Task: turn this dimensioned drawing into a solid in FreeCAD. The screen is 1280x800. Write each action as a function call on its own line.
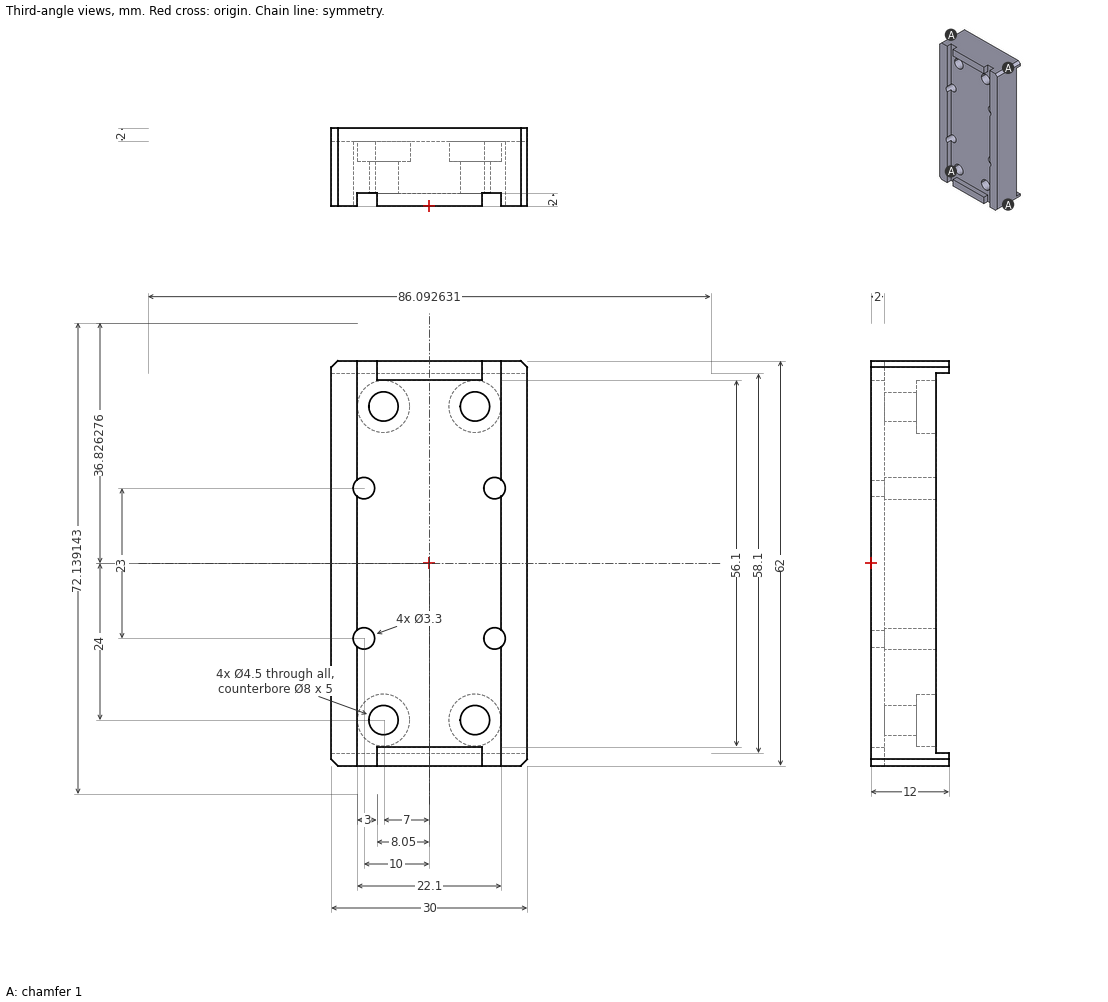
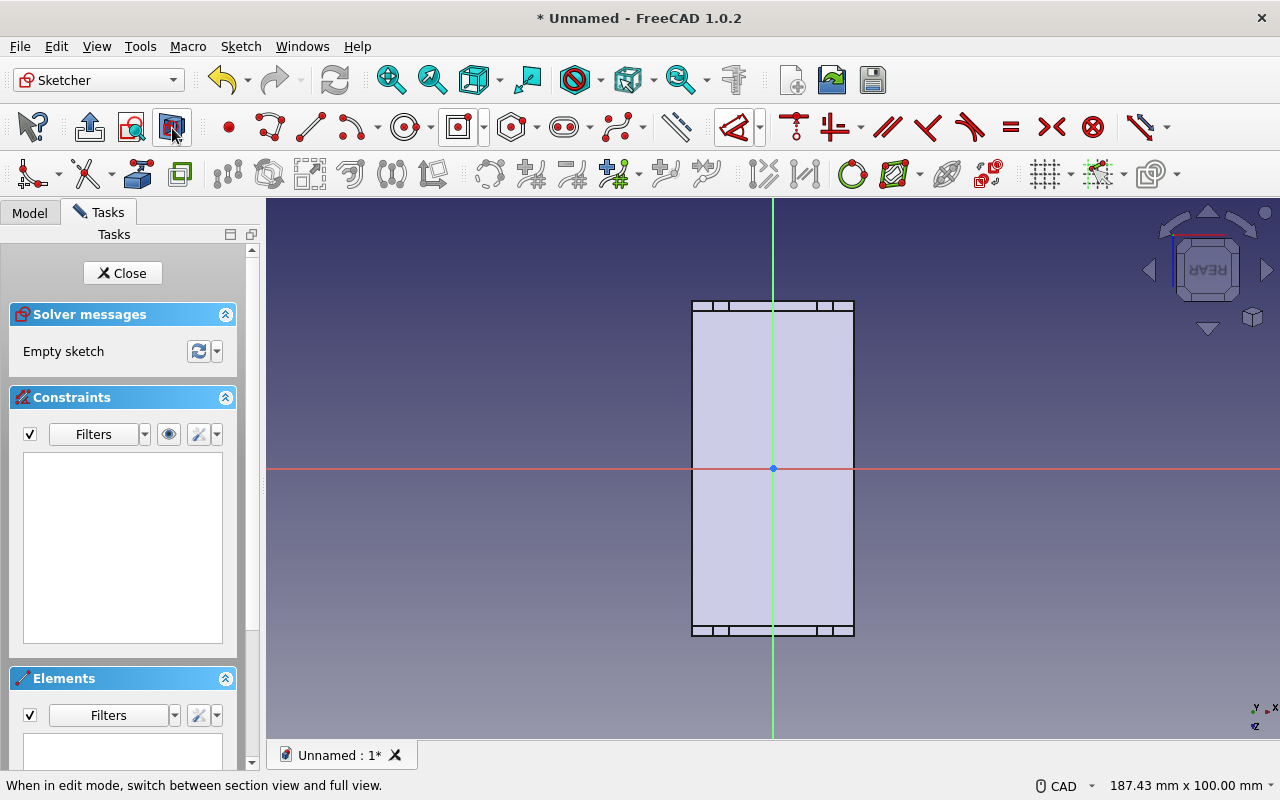
scroll(829, 468, up, 4)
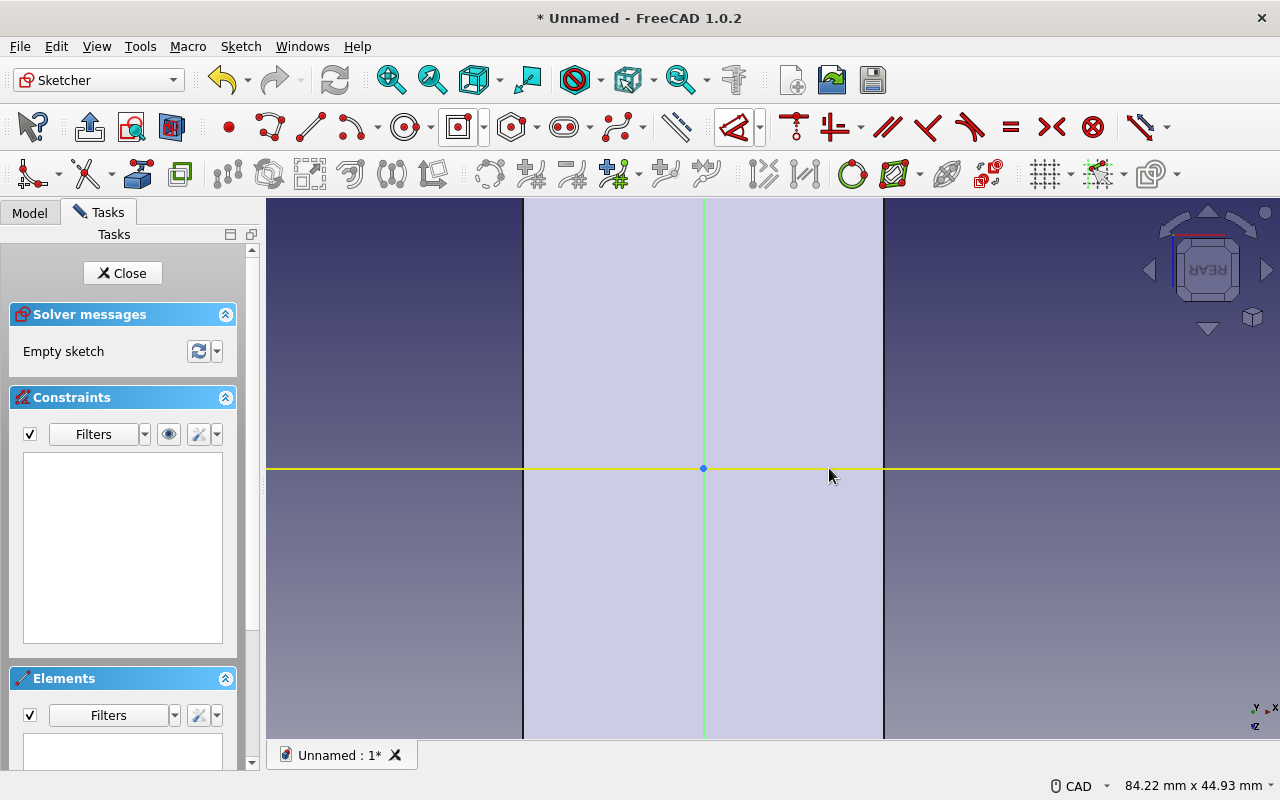
click(404, 128)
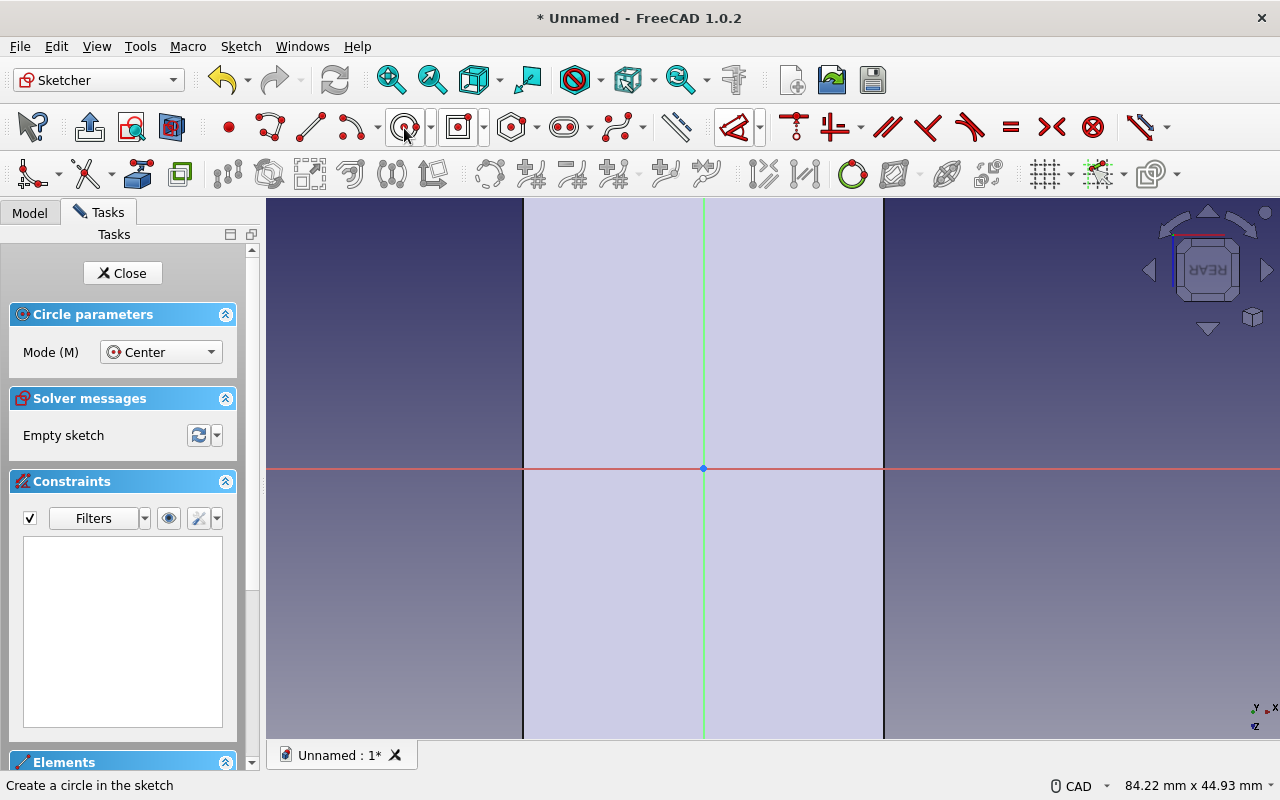
click(583, 330)
click(597, 316)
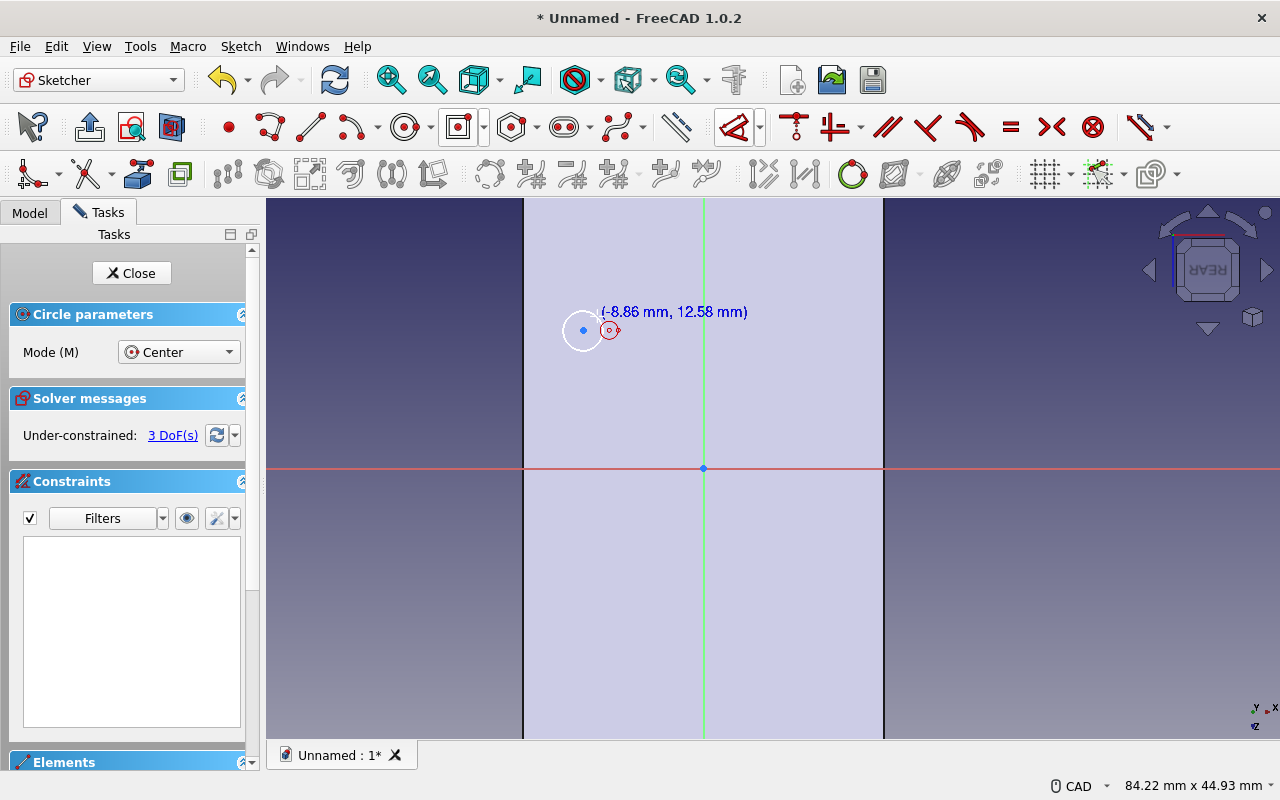
click(824, 330)
click(838, 316)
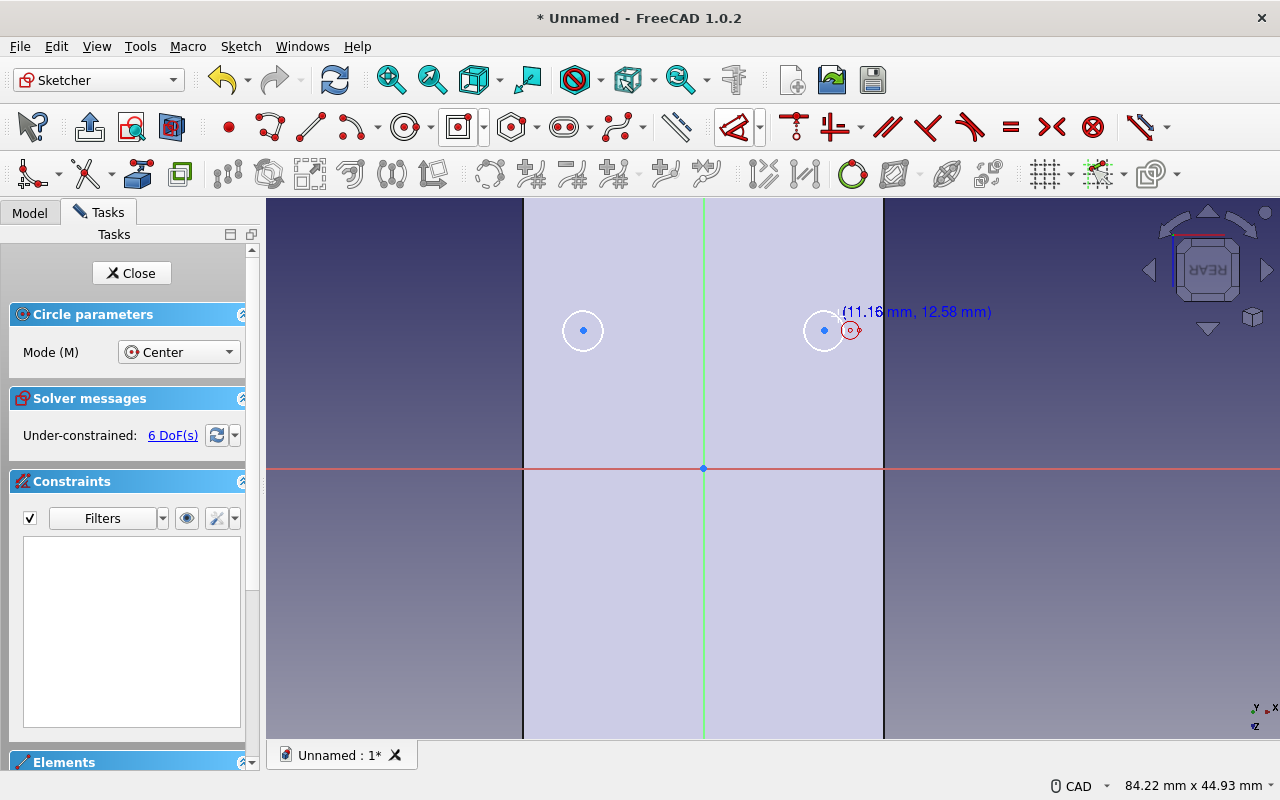
click(583, 607)
click(597, 593)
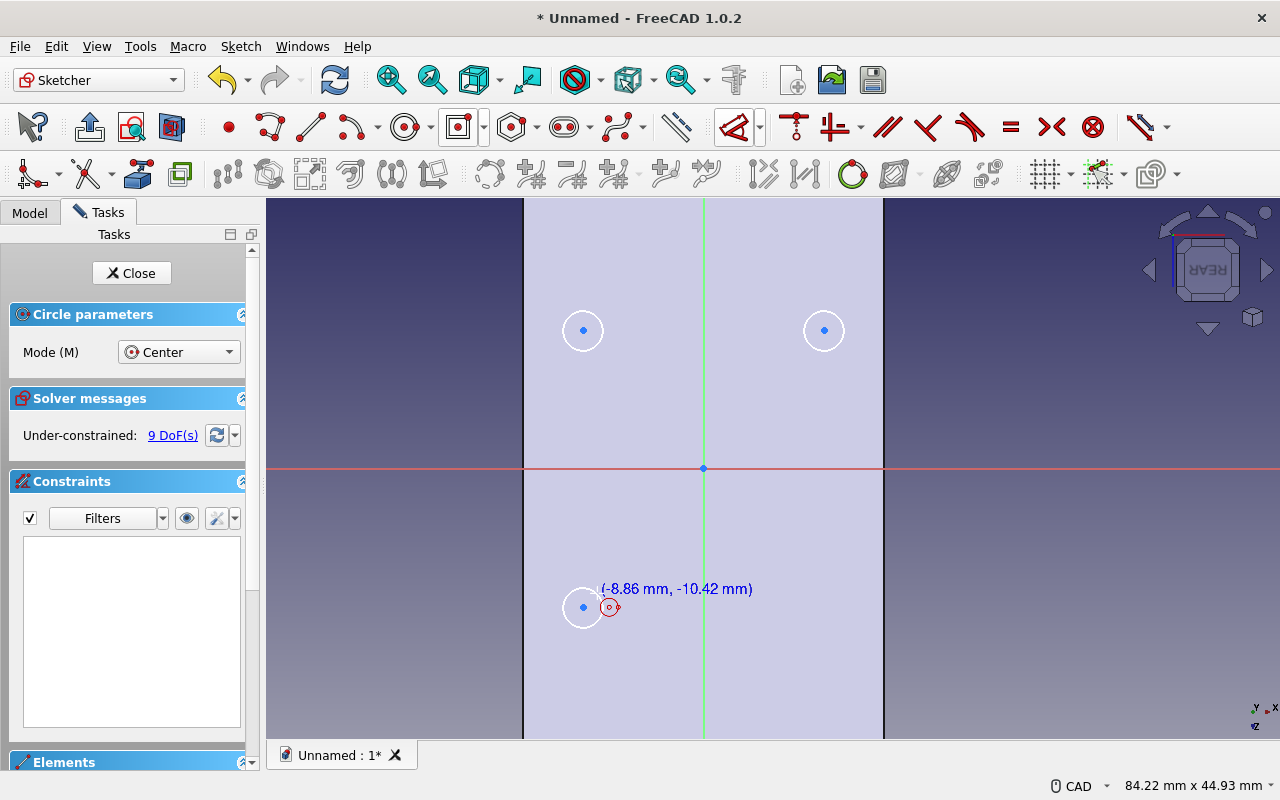
click(824, 607)
click(838, 593)
key(Escape)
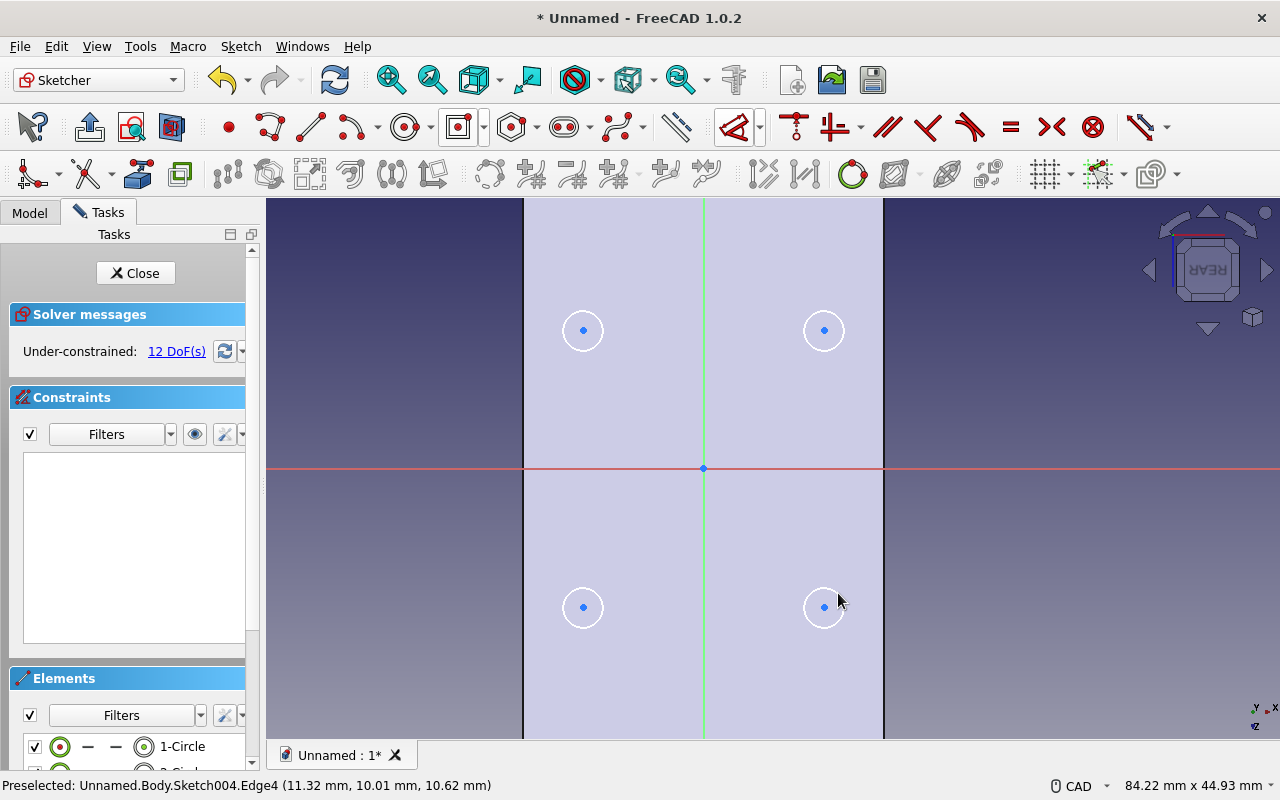
click(597, 317)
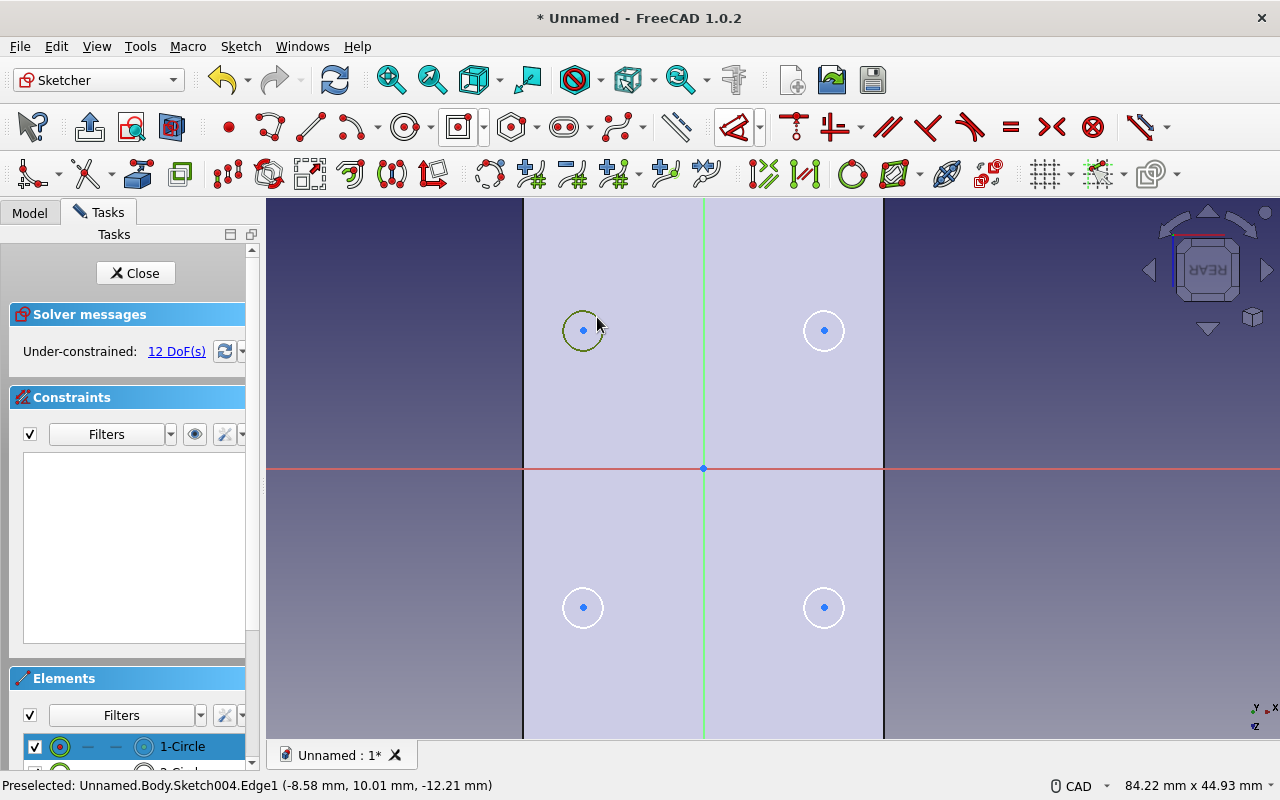
click(838, 317)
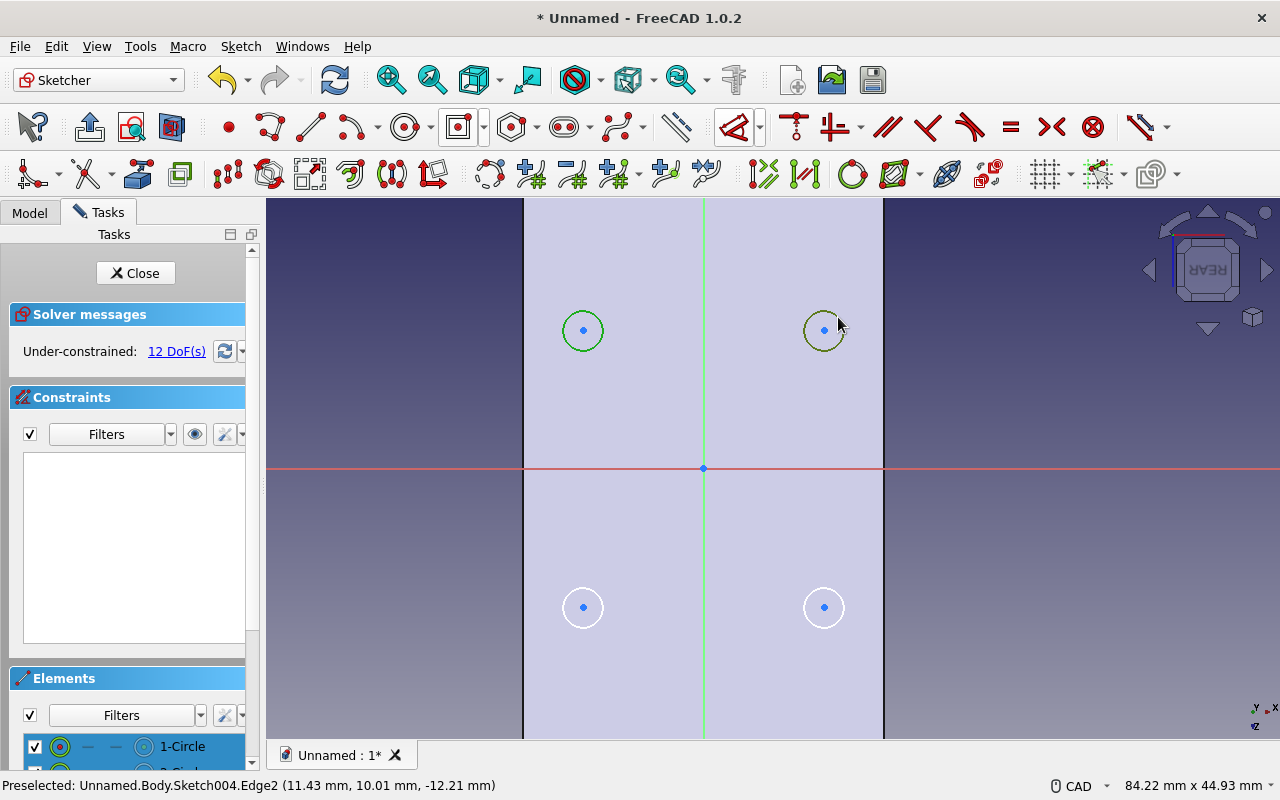
click(597, 594)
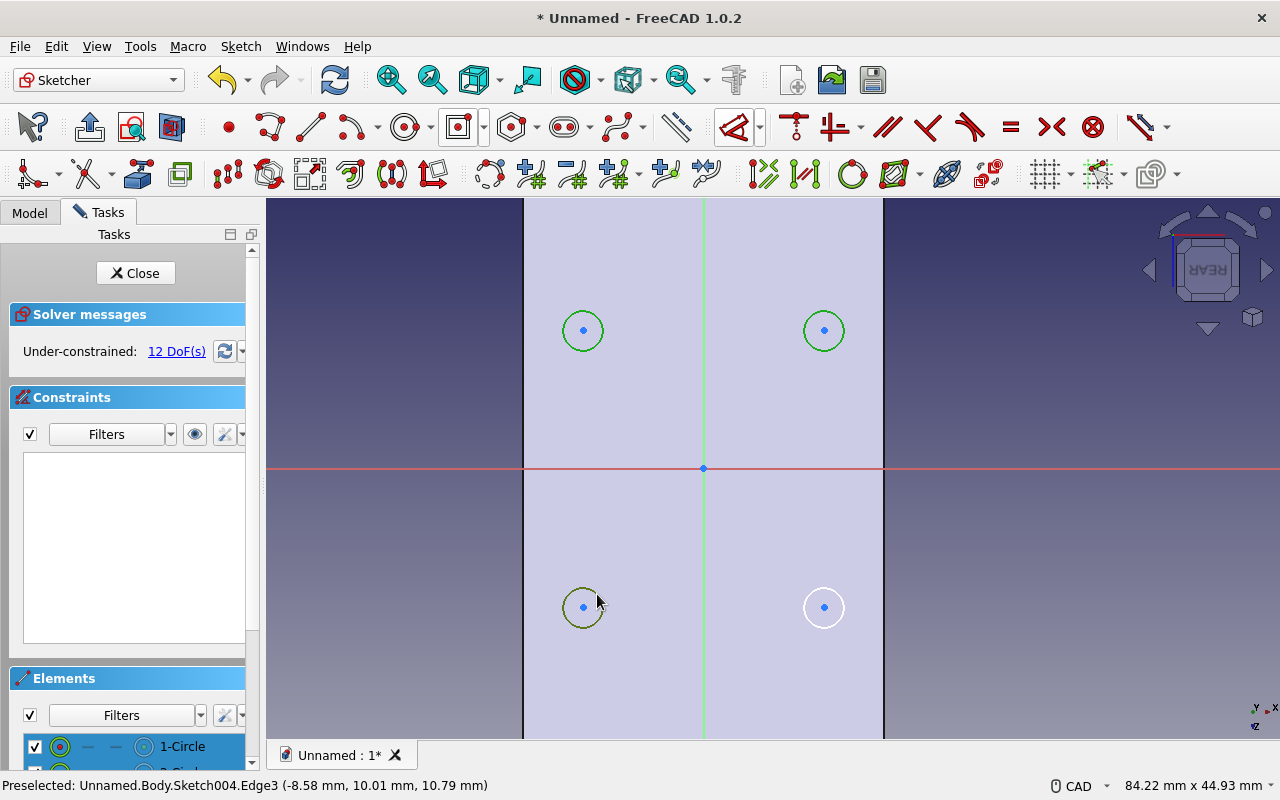
click(838, 594)